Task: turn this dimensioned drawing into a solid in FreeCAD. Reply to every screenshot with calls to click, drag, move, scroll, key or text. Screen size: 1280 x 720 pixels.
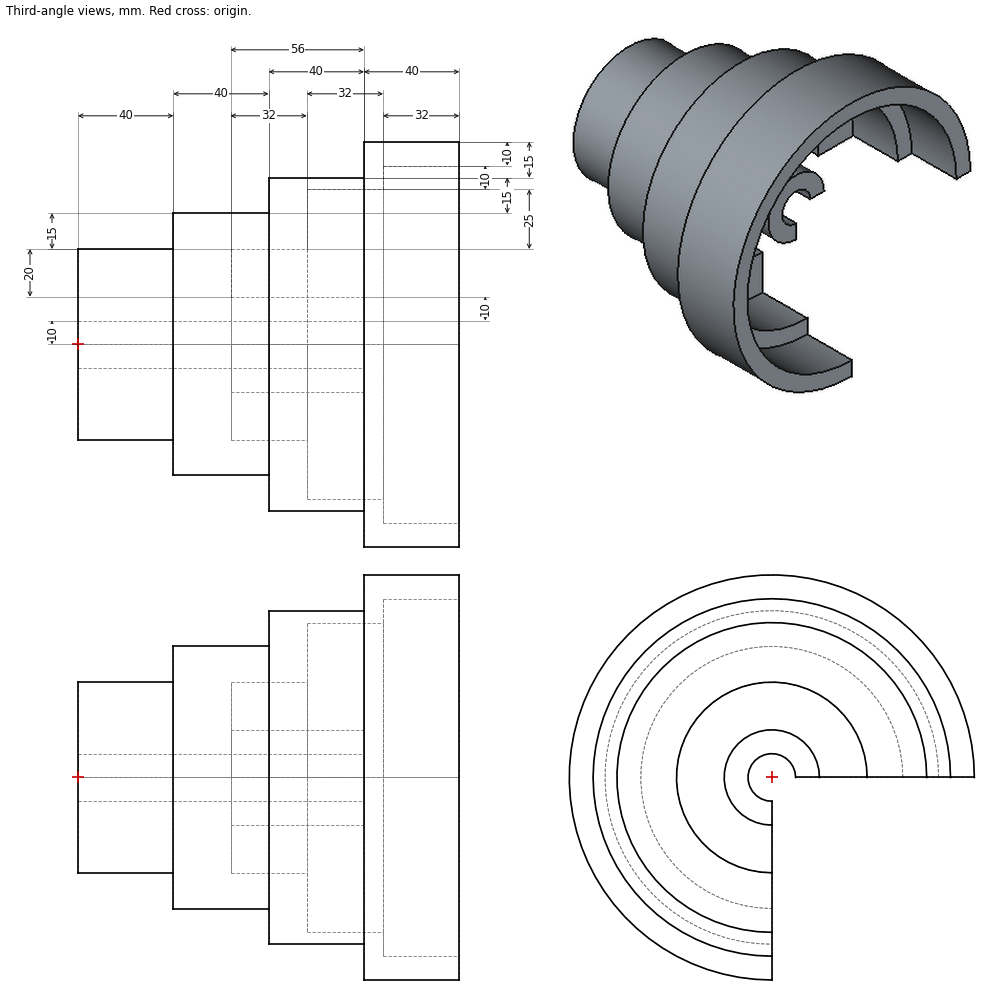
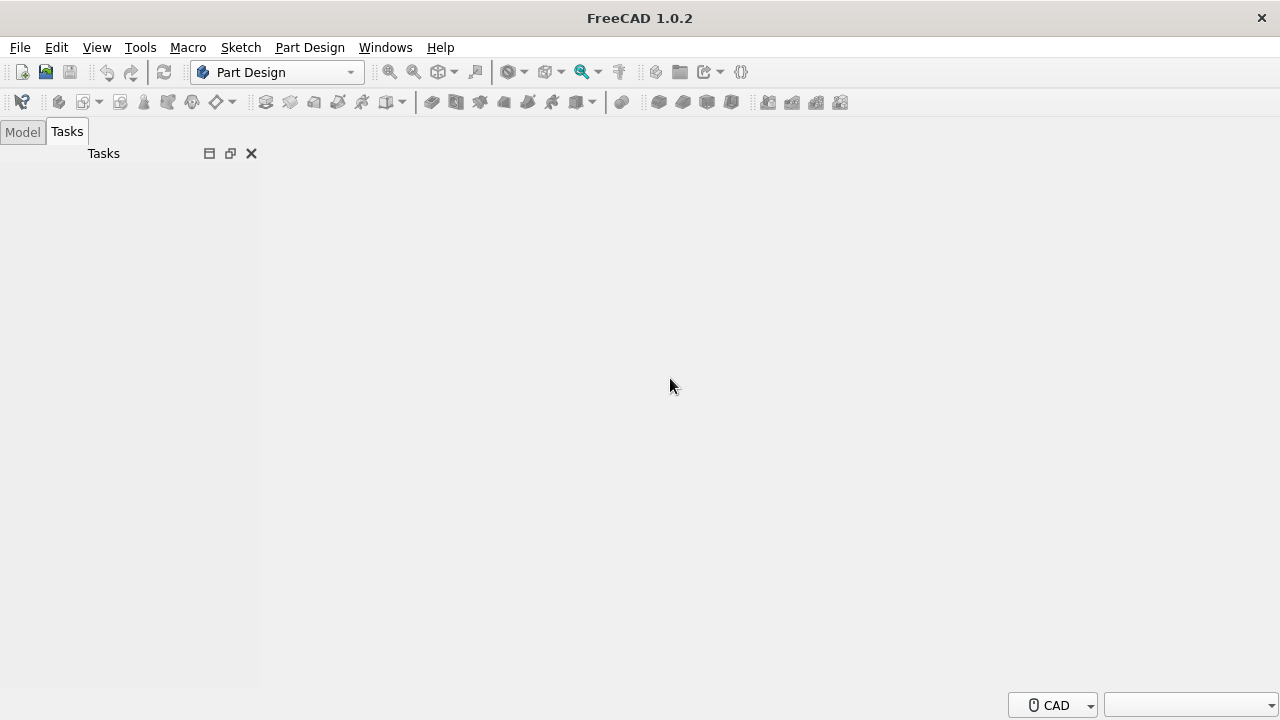
key(ctrl+n)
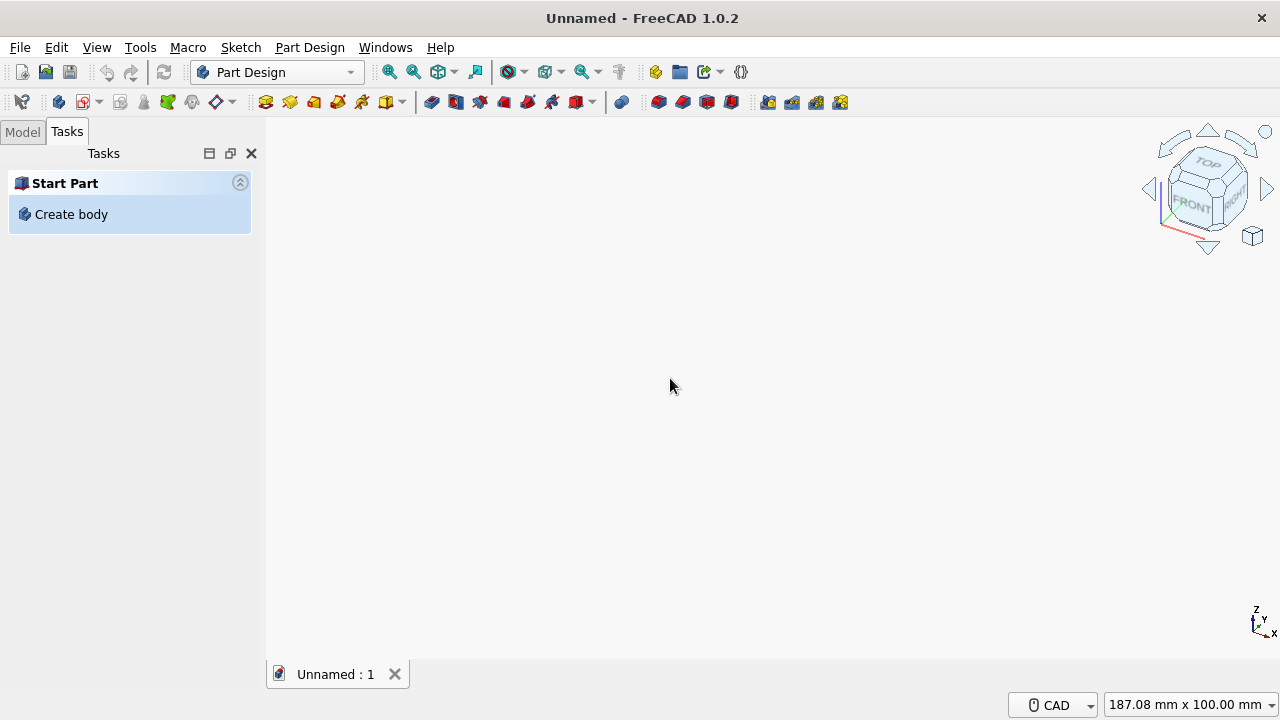
click(84, 102)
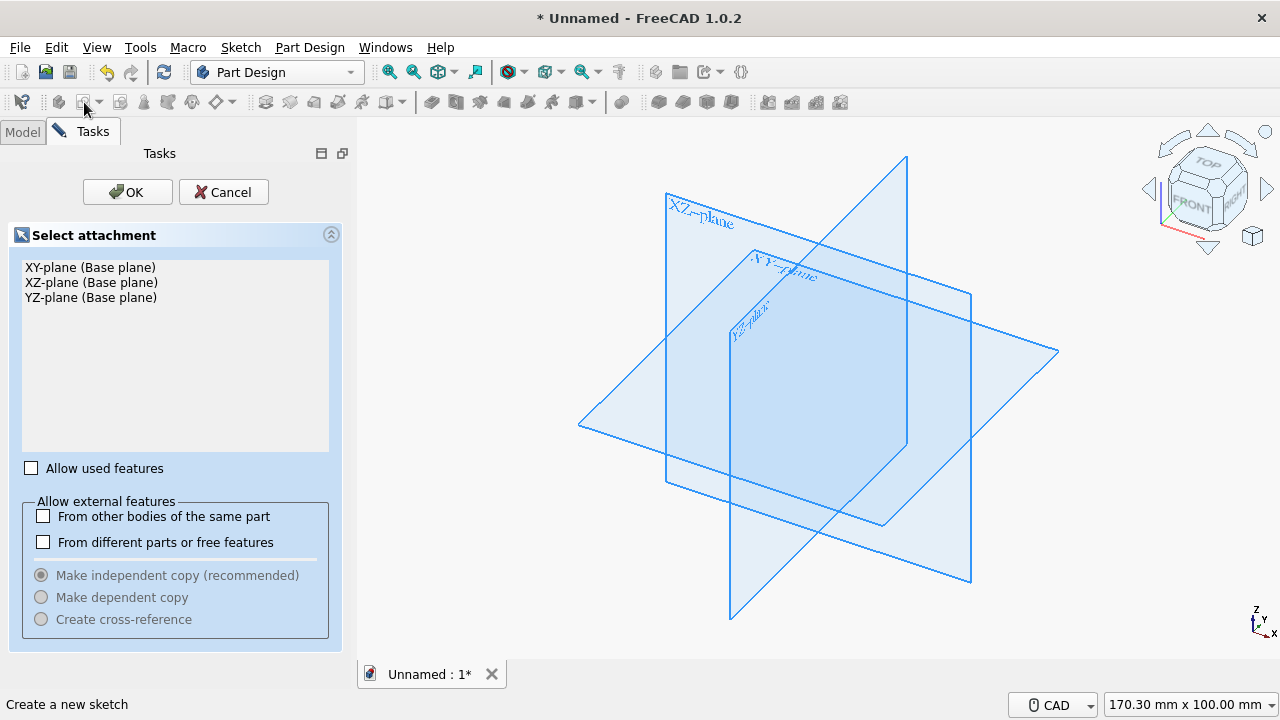
click(82, 268)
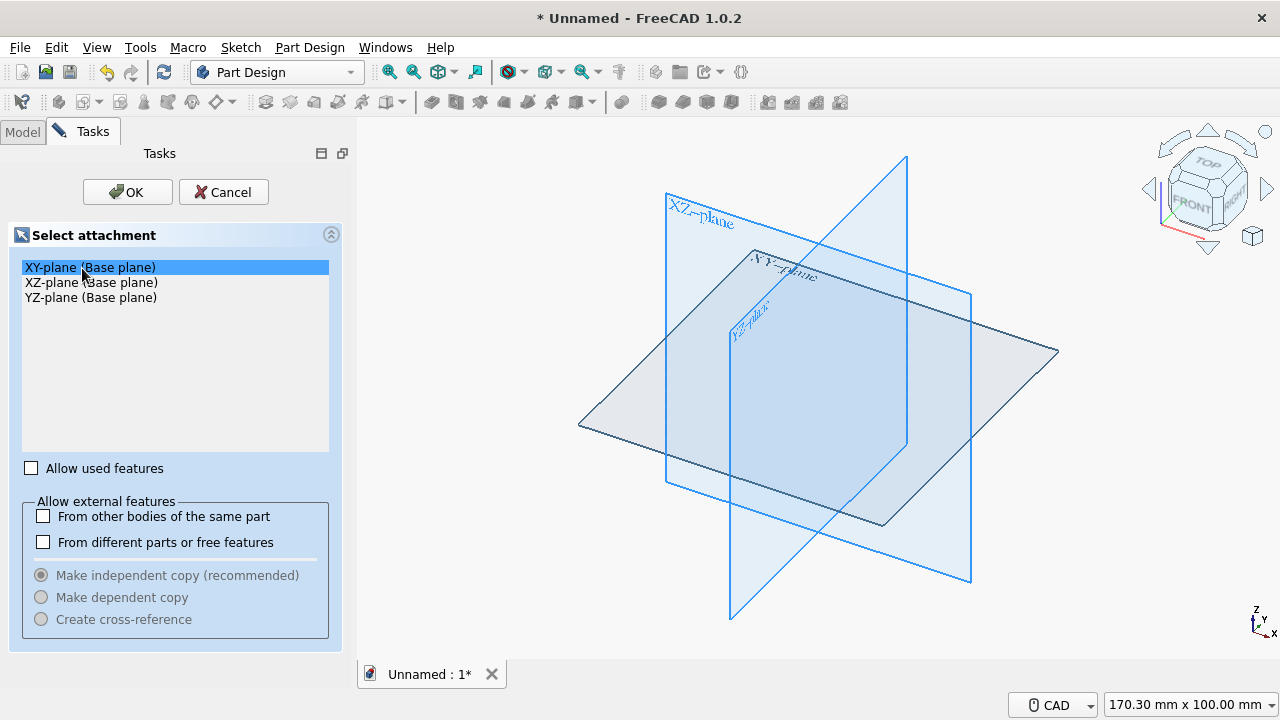
click(128, 192)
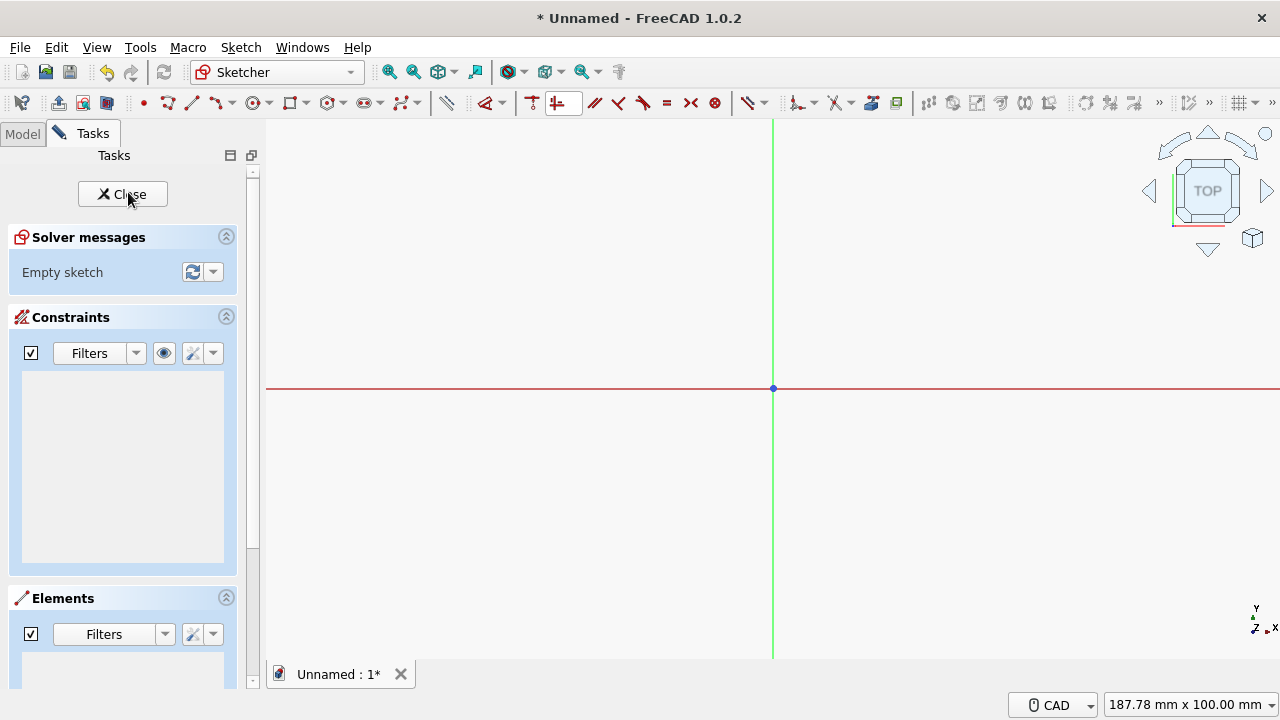
scroll(294, 631, down, 3)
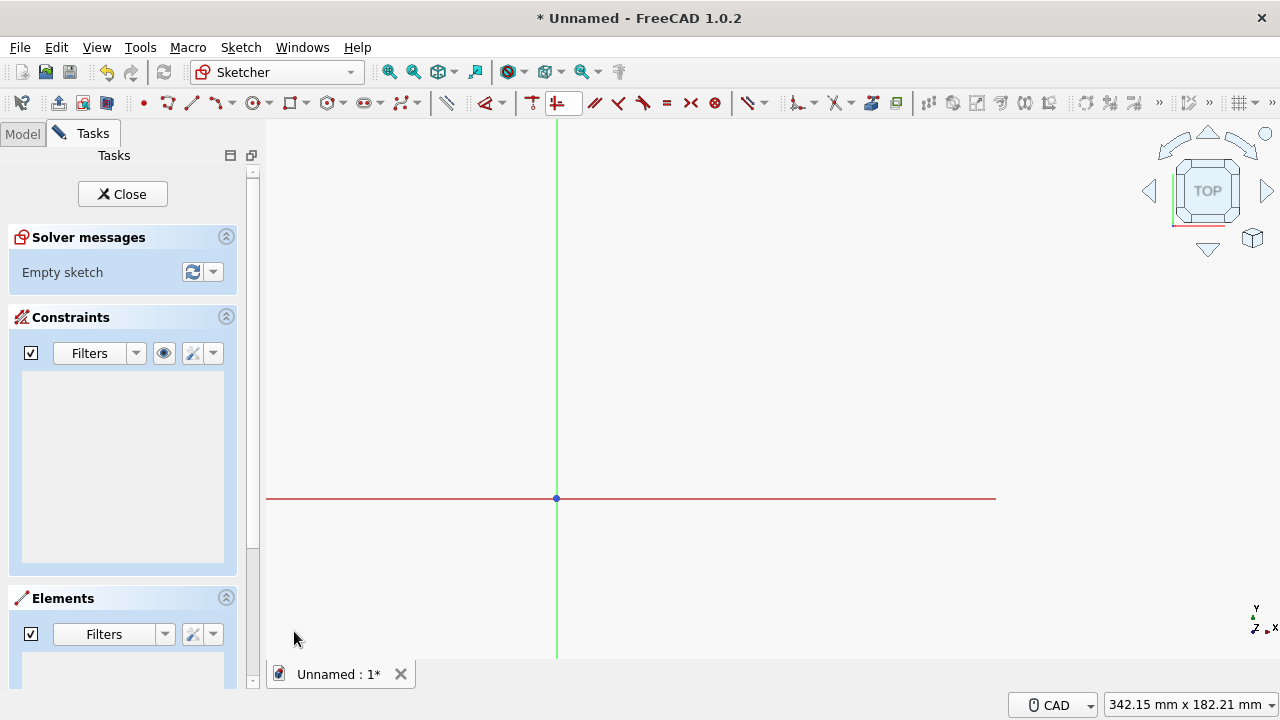
key(g)
key(m)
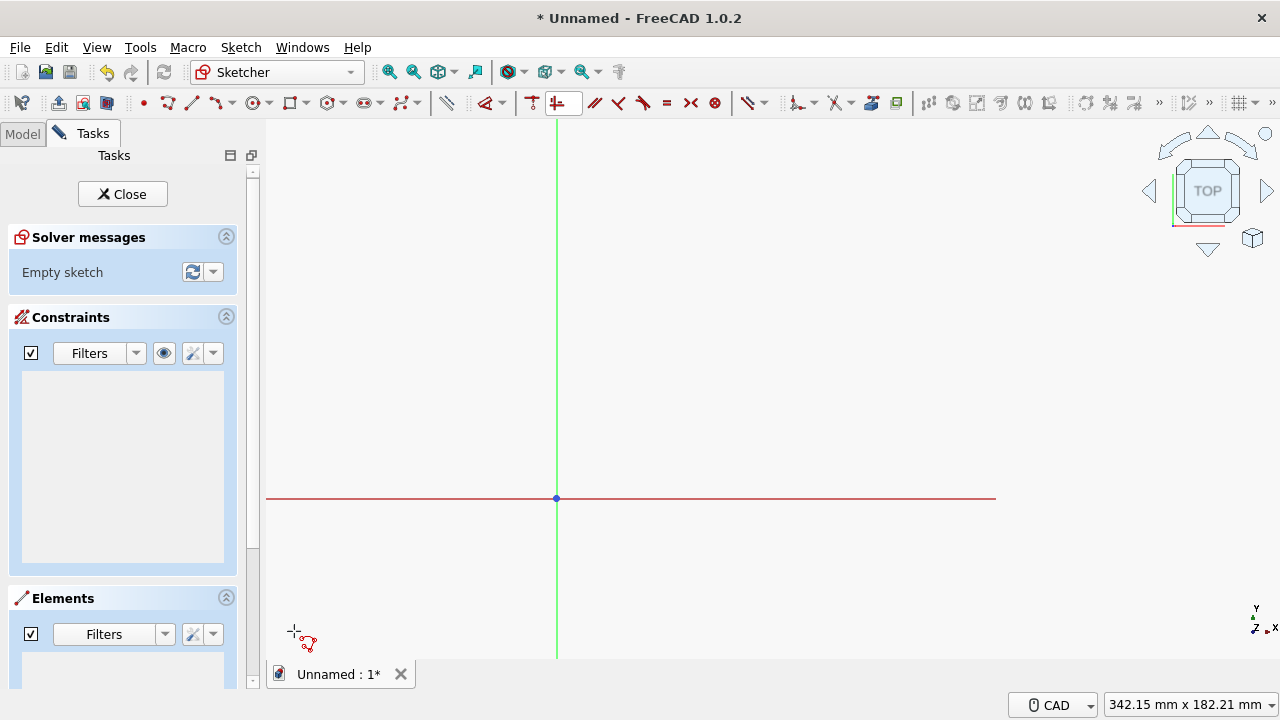
click(557, 469)
click(913, 469)
click(913, 439)
click(747, 439)
click(747, 380)
click(841, 380)
click(841, 306)
click(936, 306)
click(936, 276)
click(1031, 276)
click(1031, 247)
click(913, 247)
click(913, 291)
click(794, 291)
click(794, 336)
click(675, 336)
click(675, 380)
click(566, 380)
click(557, 470)
key(Escape)
key(Escape)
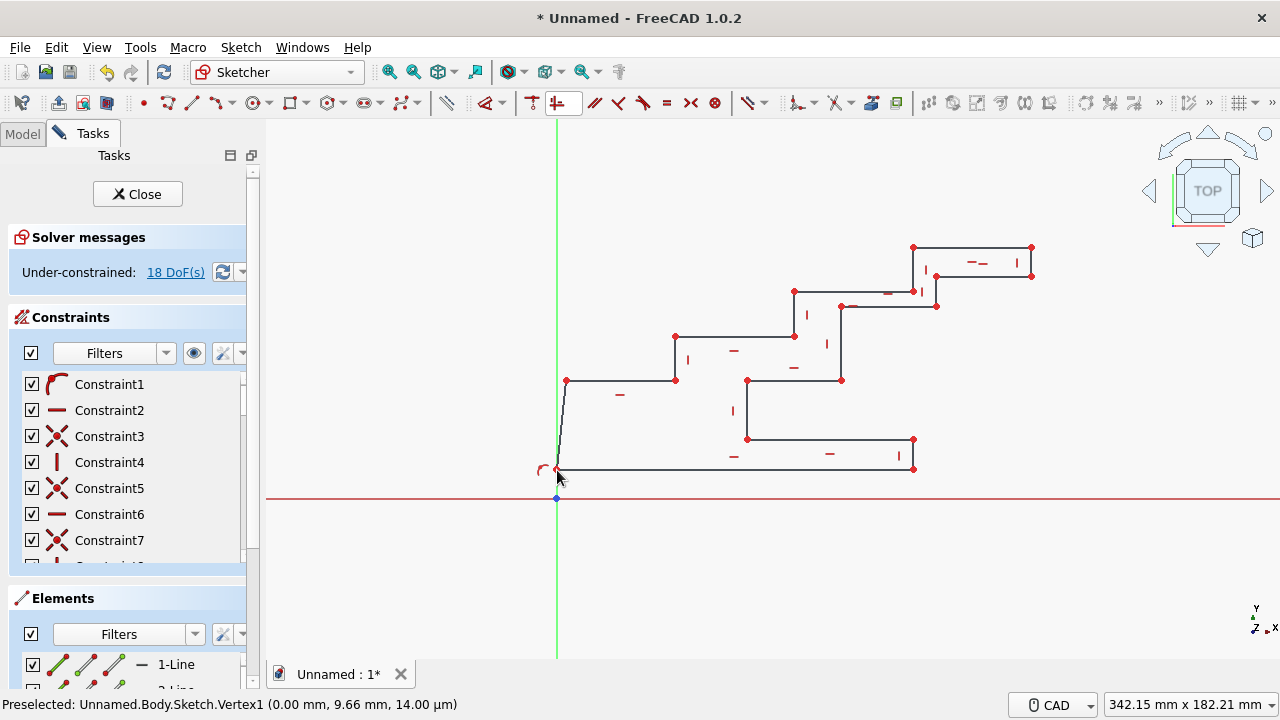
click(560, 443)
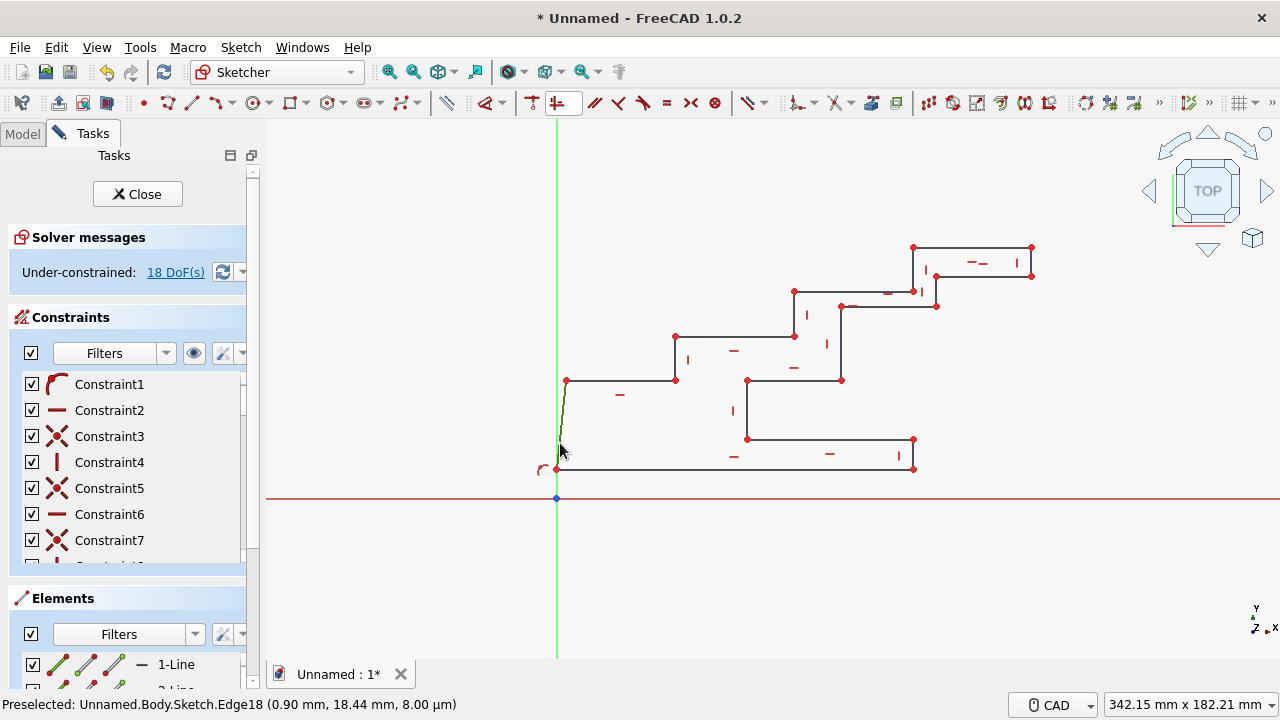
click(576, 104)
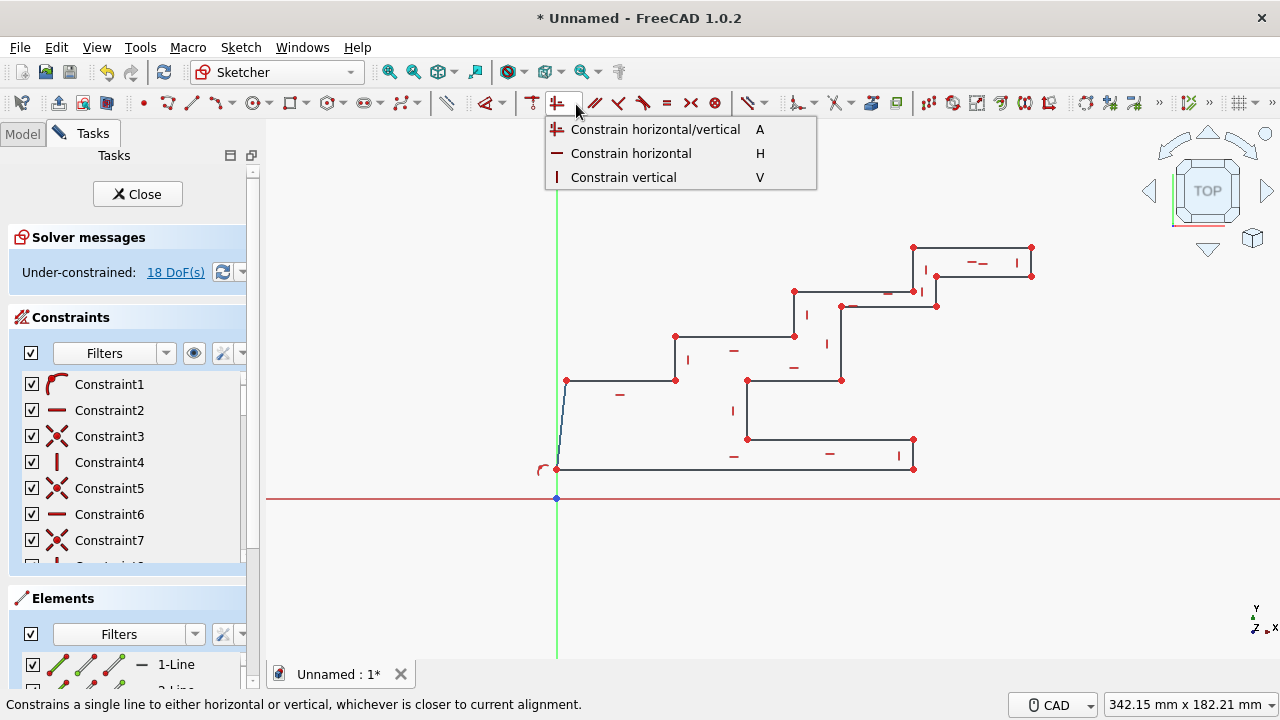
click(681, 177)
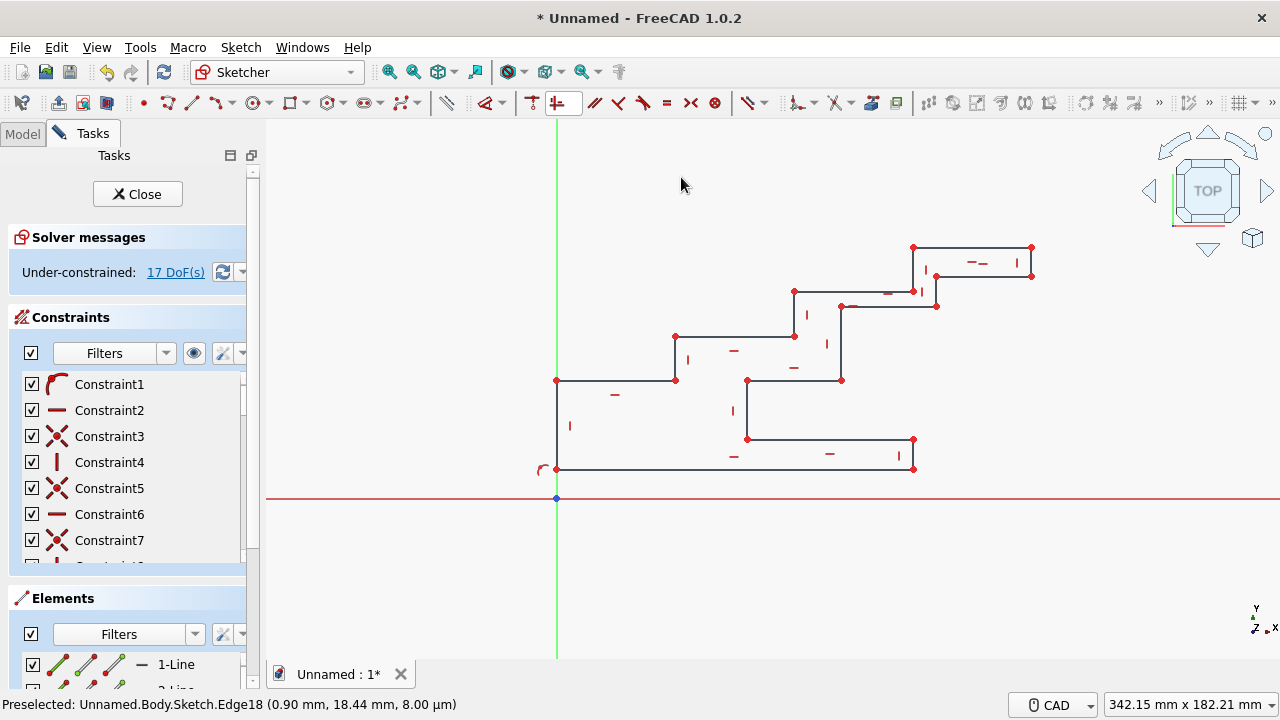
key(d)